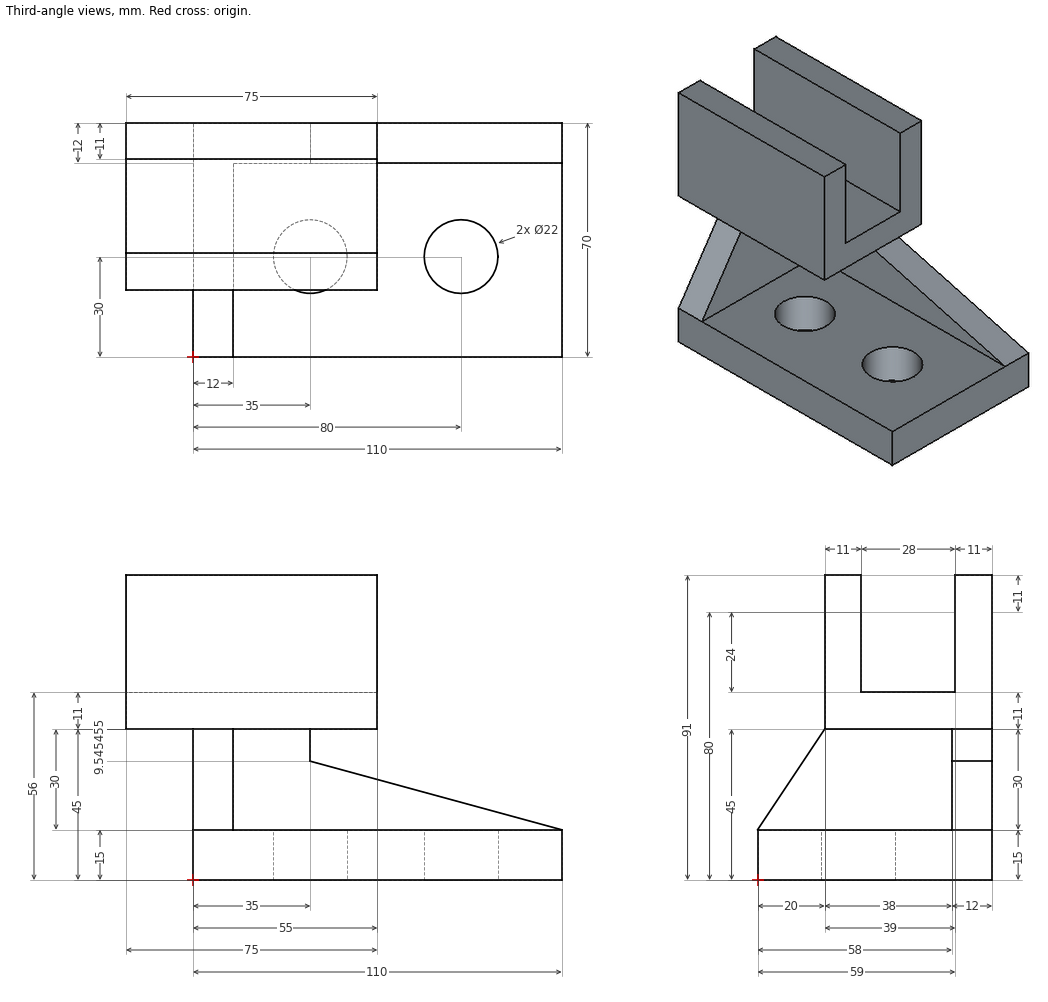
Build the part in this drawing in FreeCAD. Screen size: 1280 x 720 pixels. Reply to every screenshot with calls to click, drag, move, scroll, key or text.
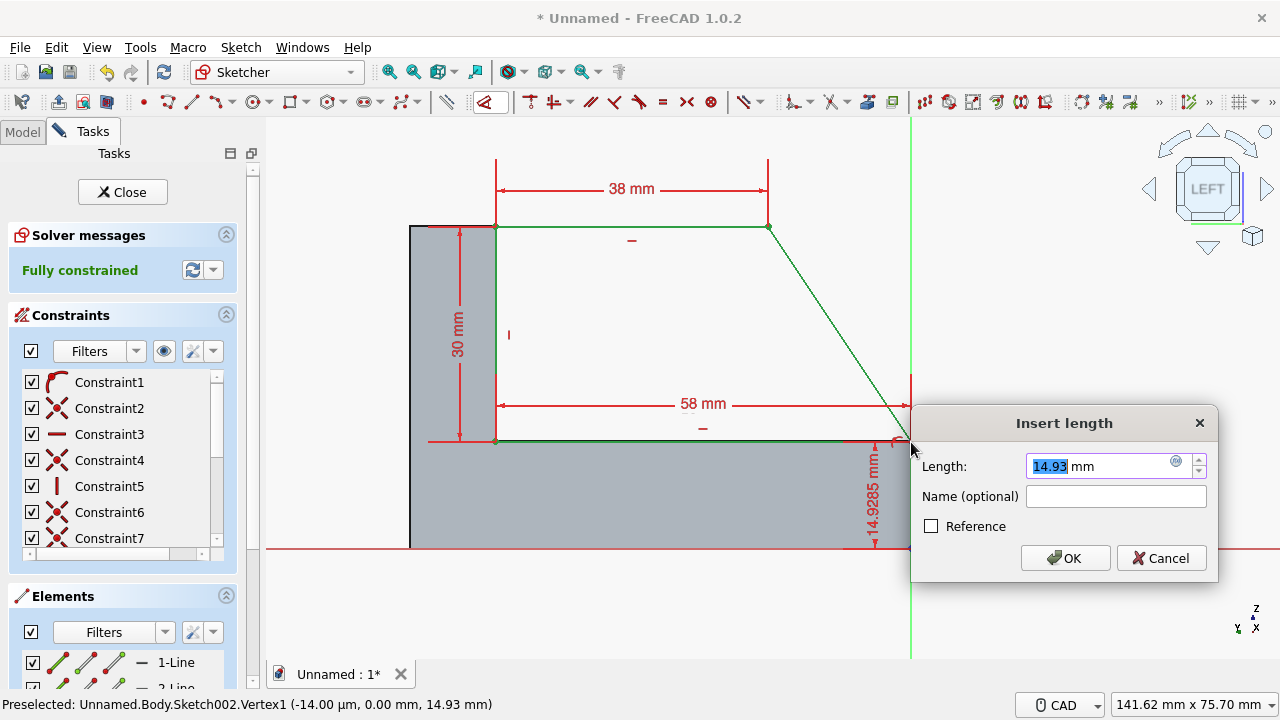
text(15)
key(Return)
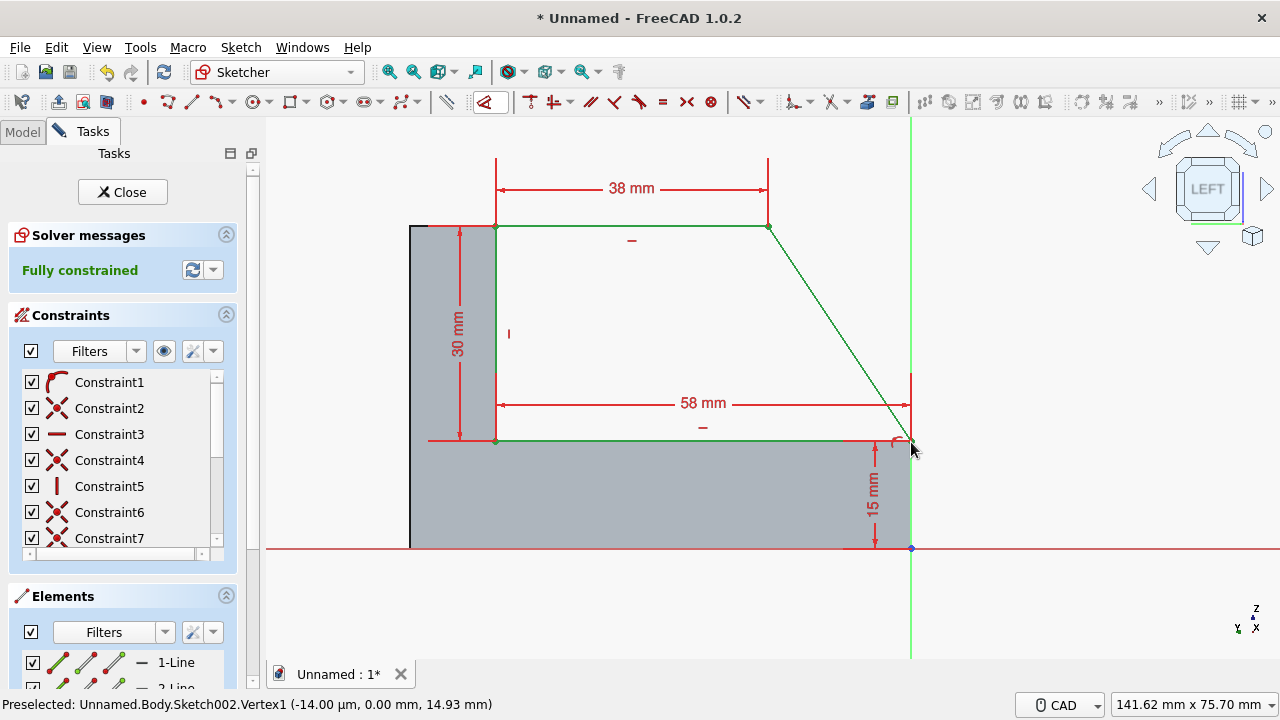
click(123, 192)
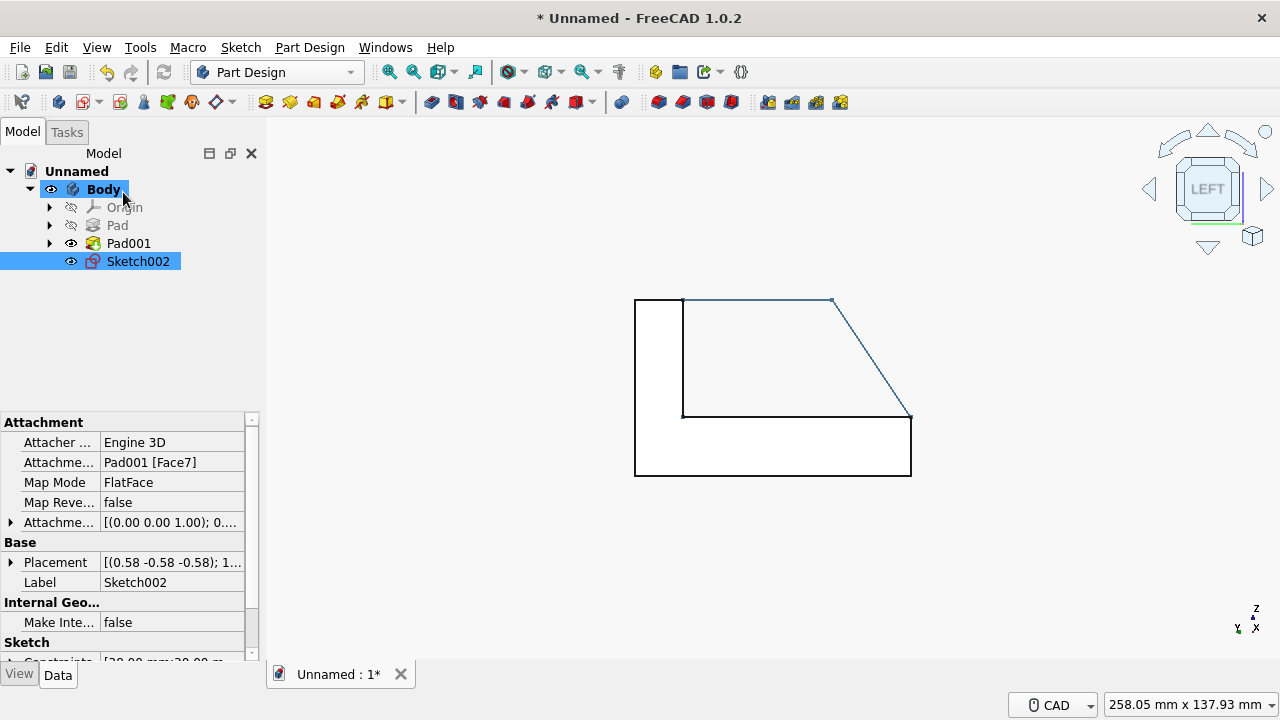
click(266, 102)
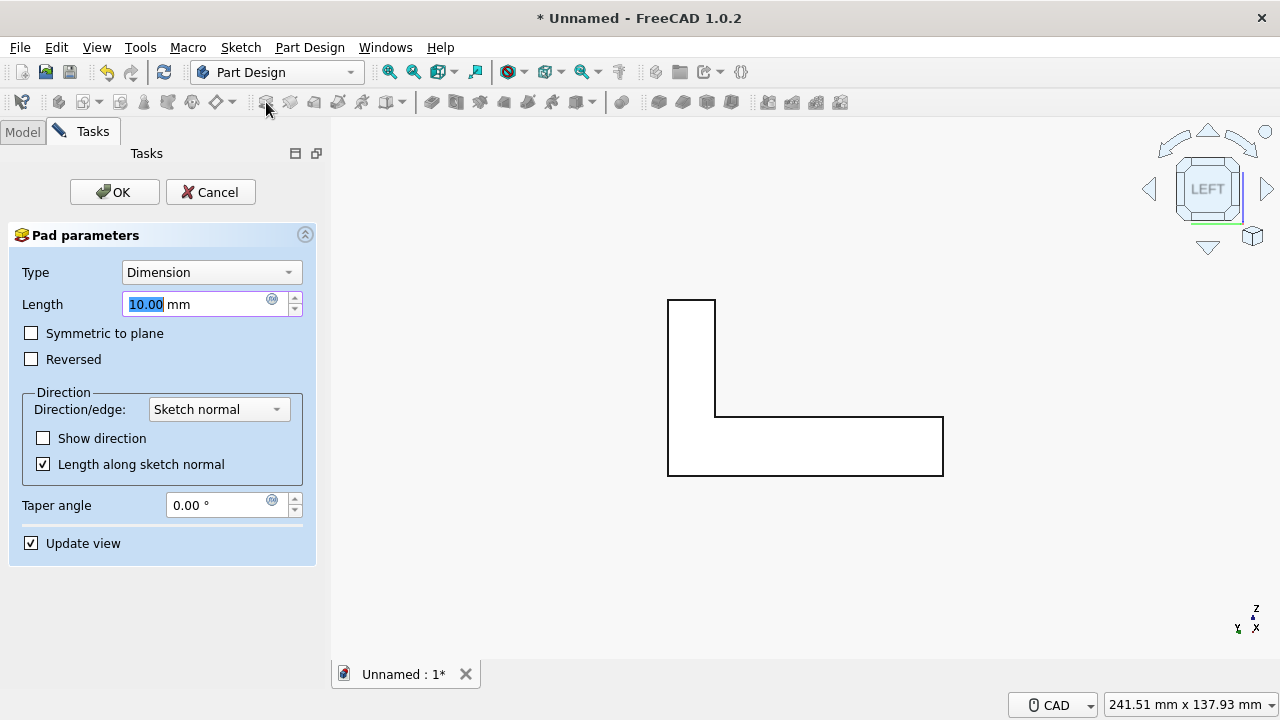
text(12)
key(Tab)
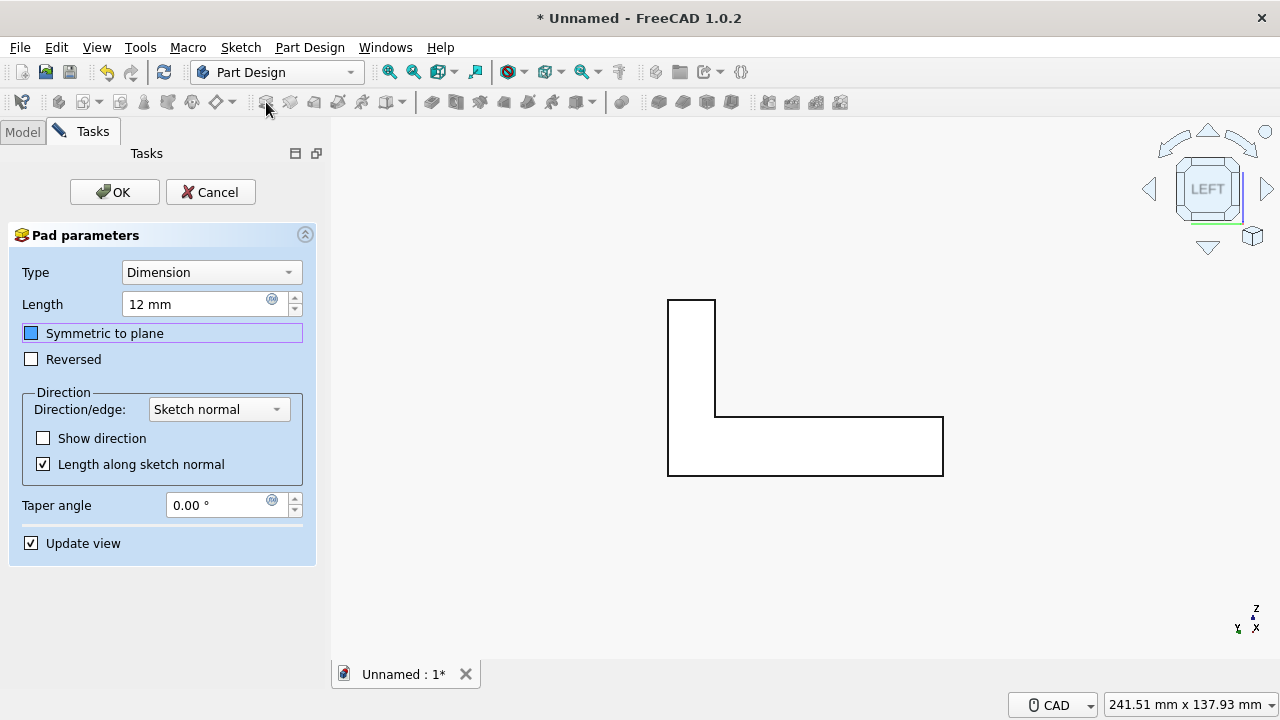
click(30, 359)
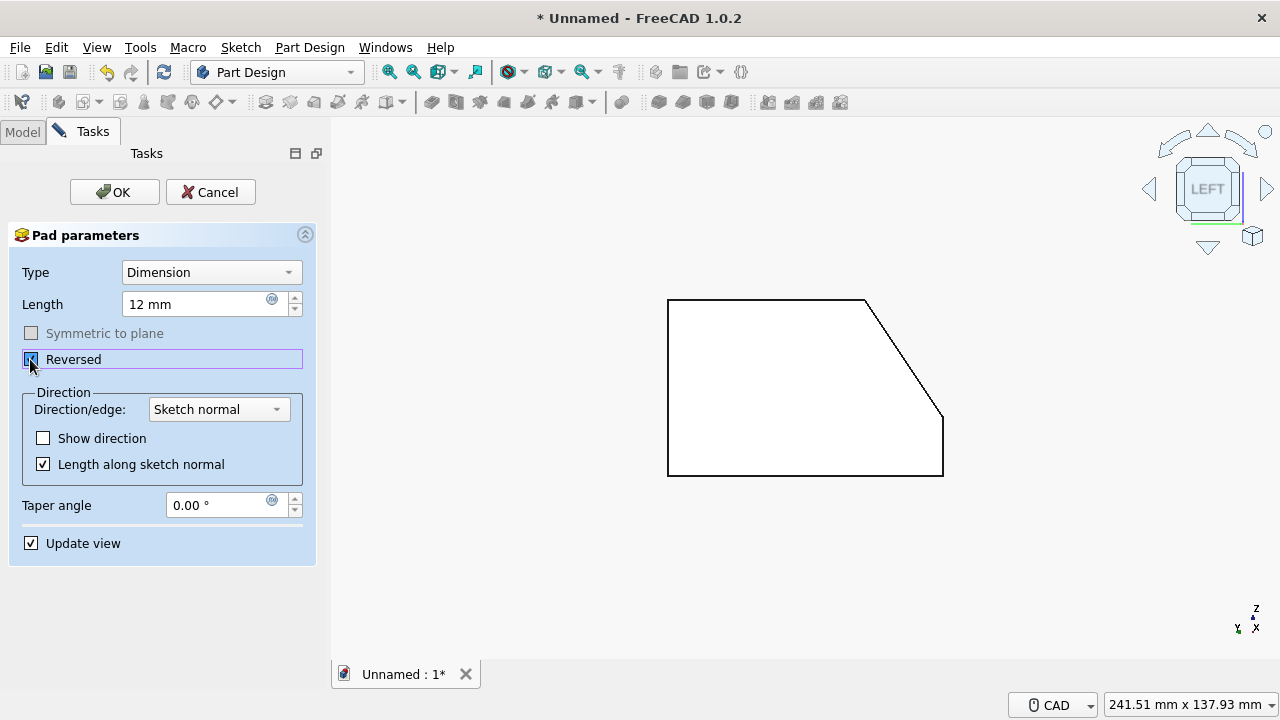
click(115, 192)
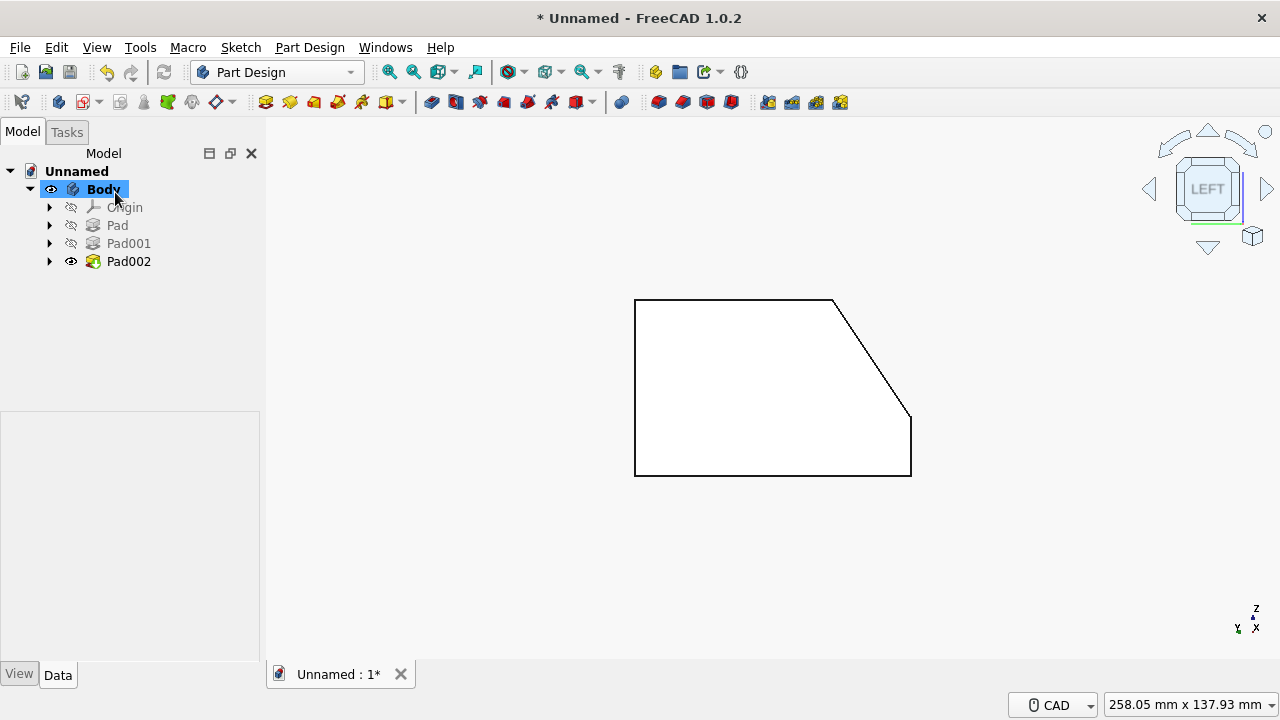
click(390, 72)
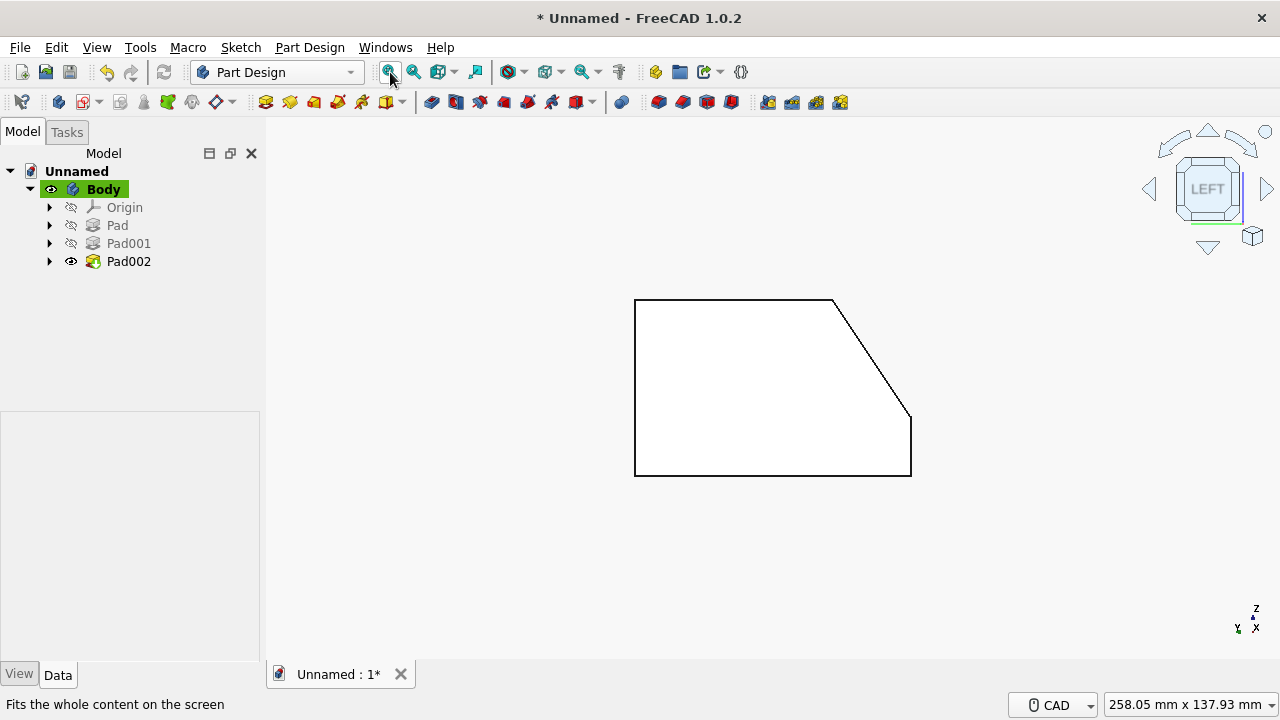
key(4)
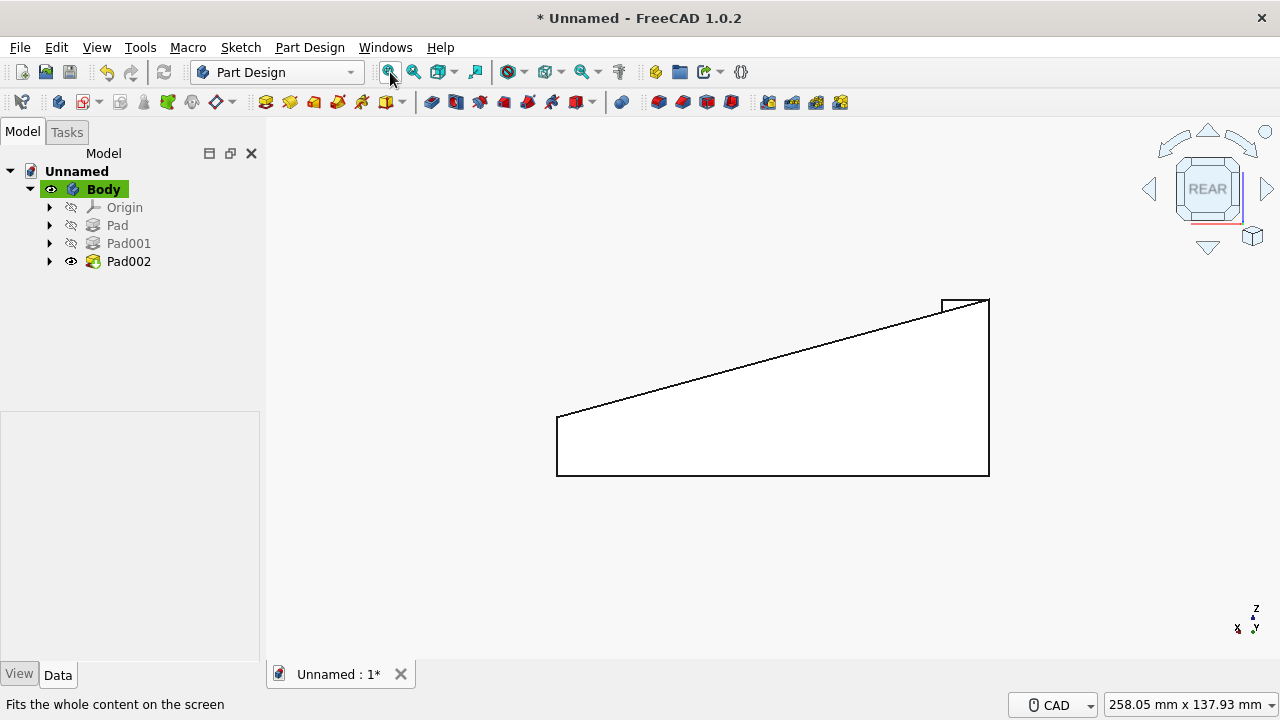
click(390, 72)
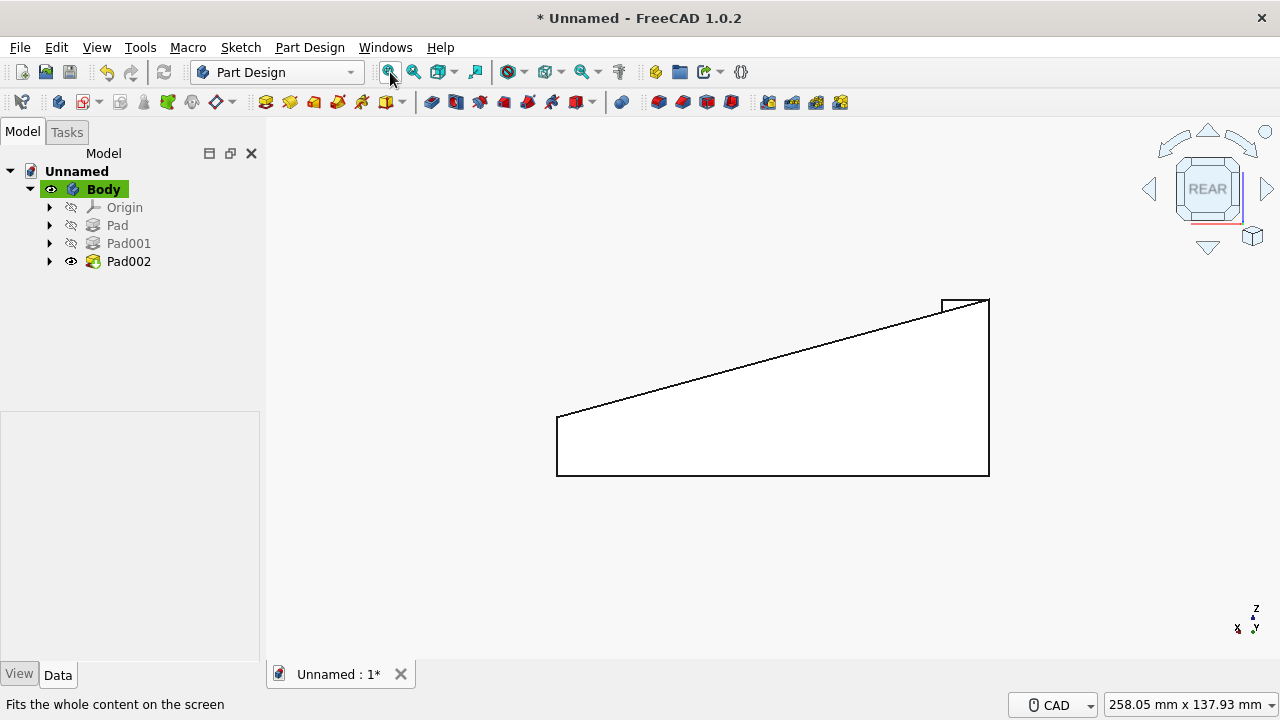
click(835, 412)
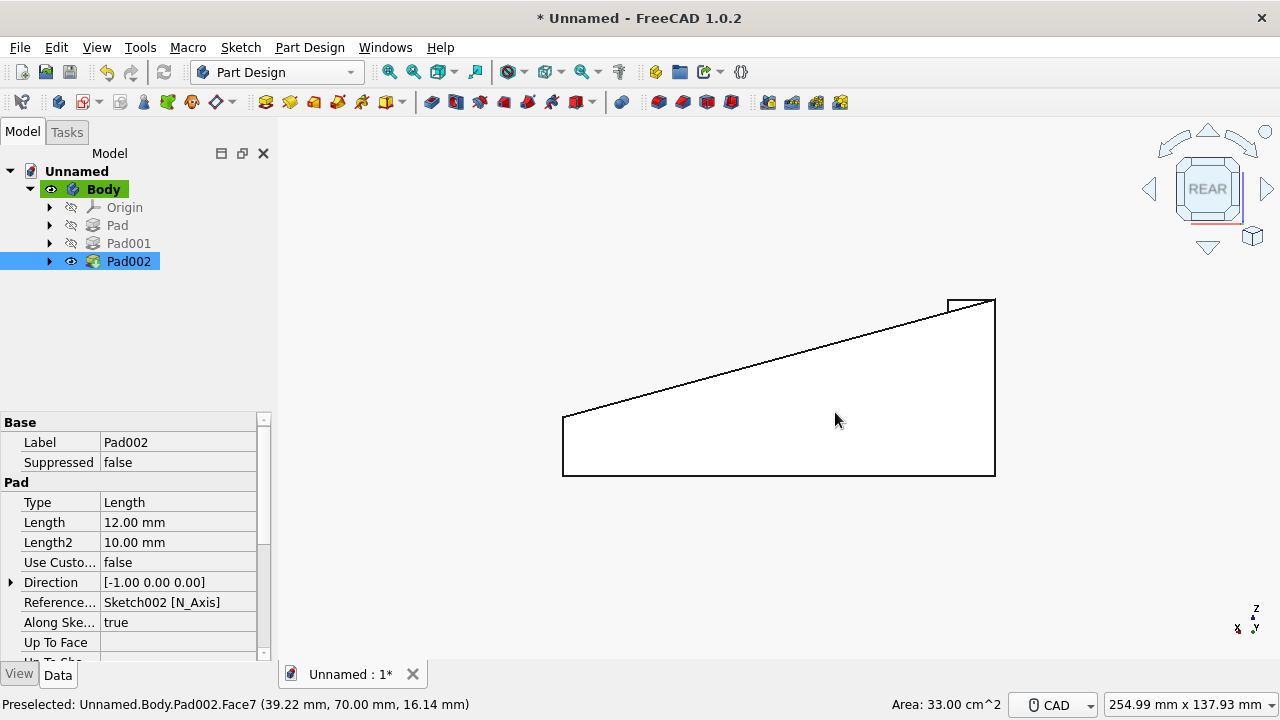
click(84, 102)